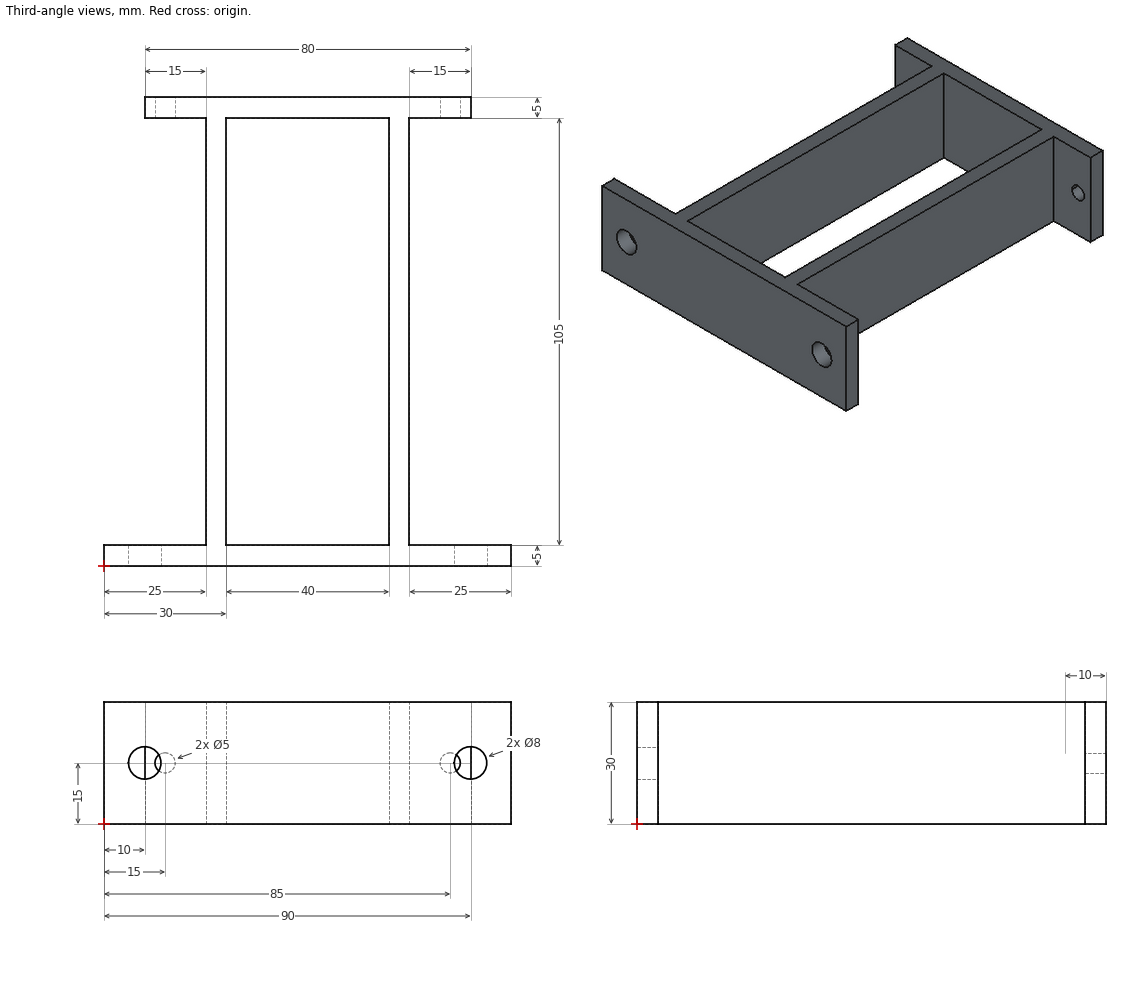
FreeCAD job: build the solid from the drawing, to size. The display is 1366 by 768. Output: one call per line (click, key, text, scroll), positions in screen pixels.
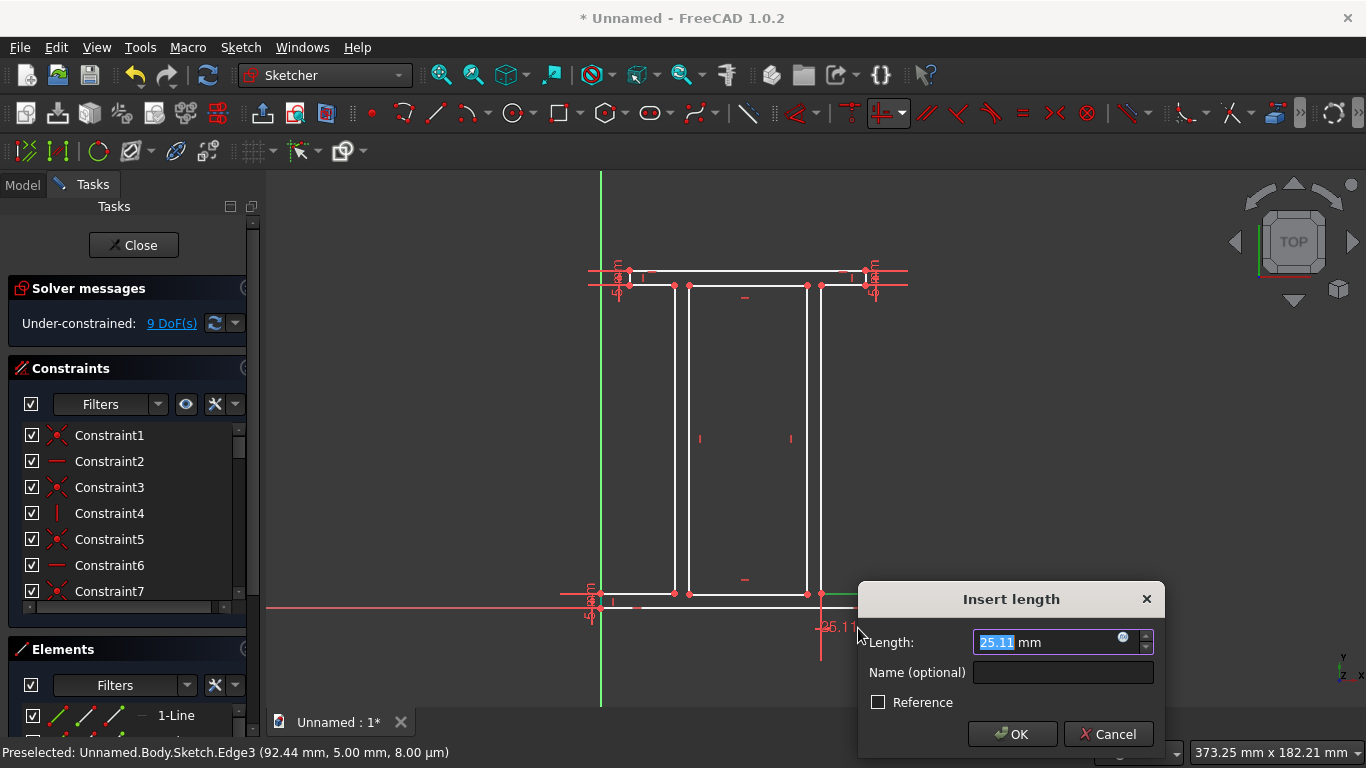
text(25)
key(Return)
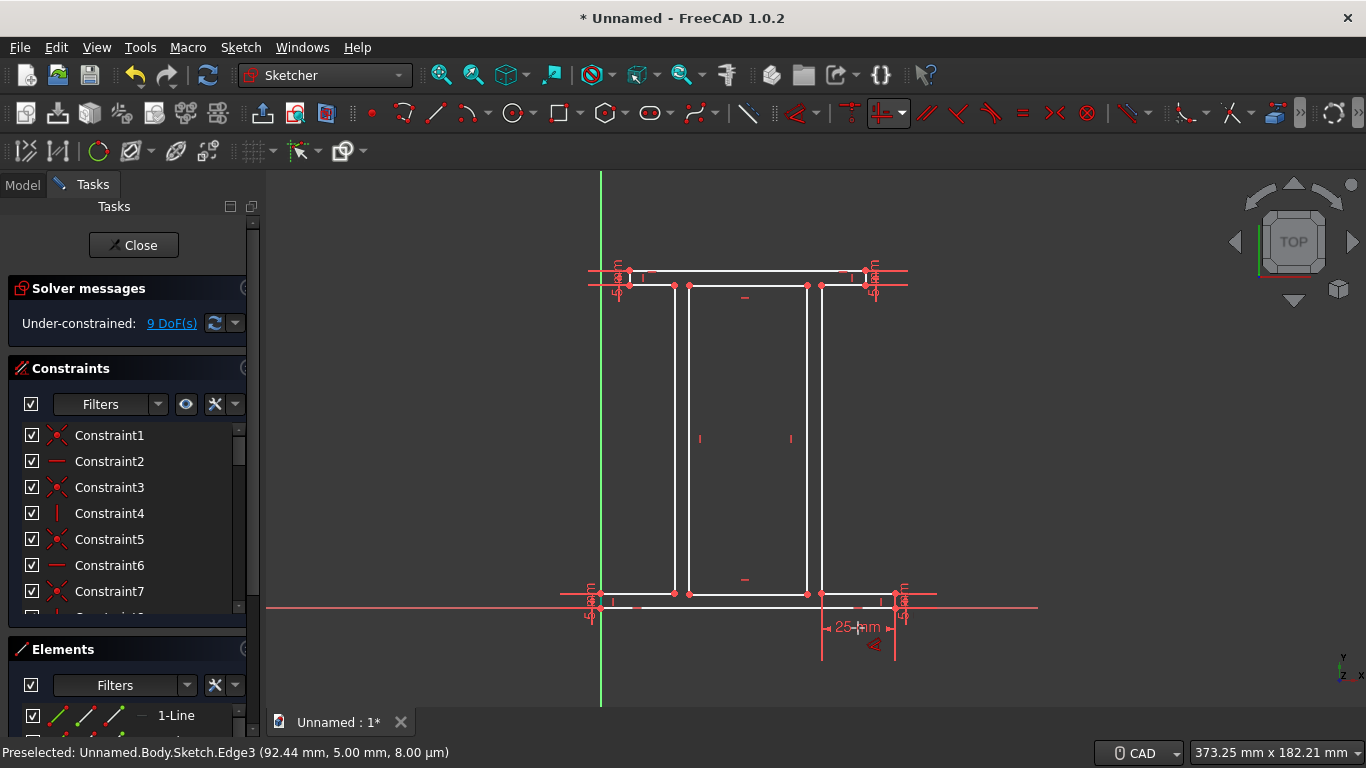
click(835, 285)
click(844, 251)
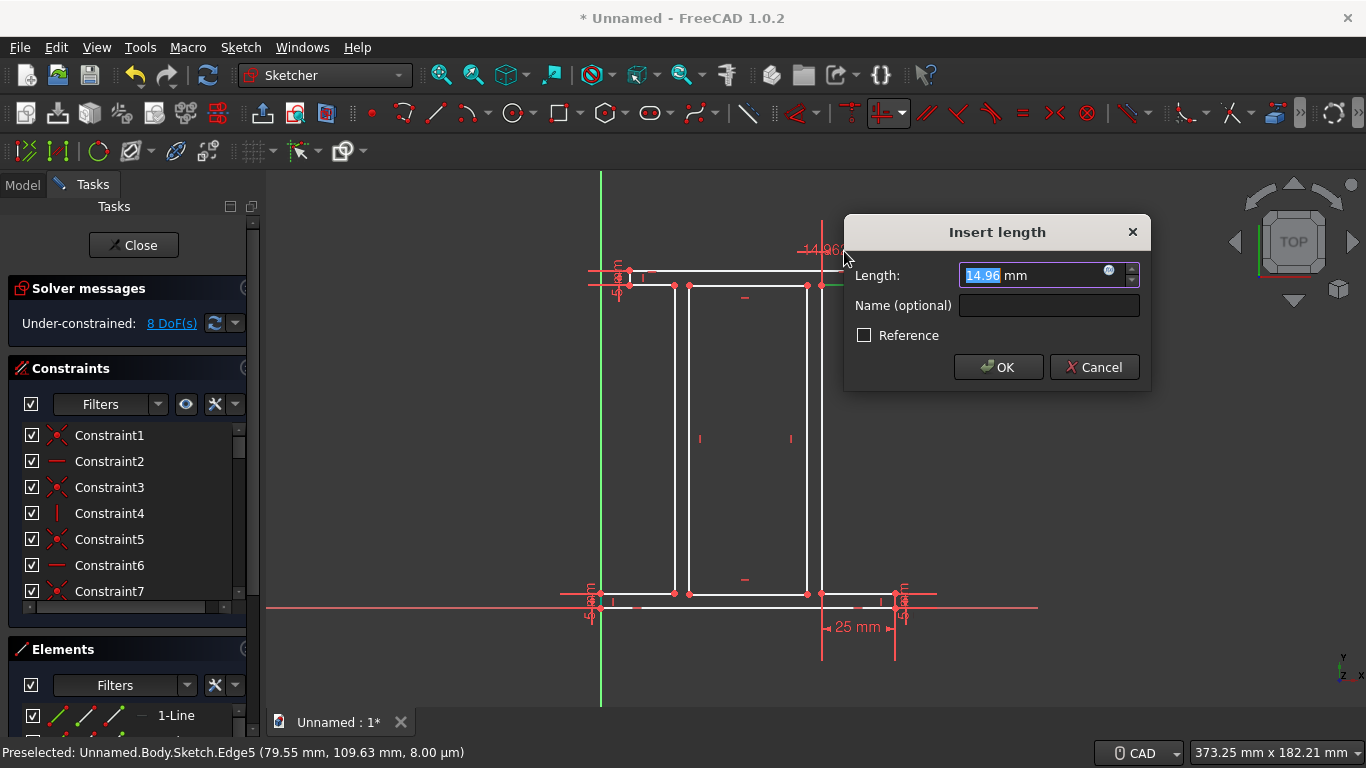
text(15)
key(Return)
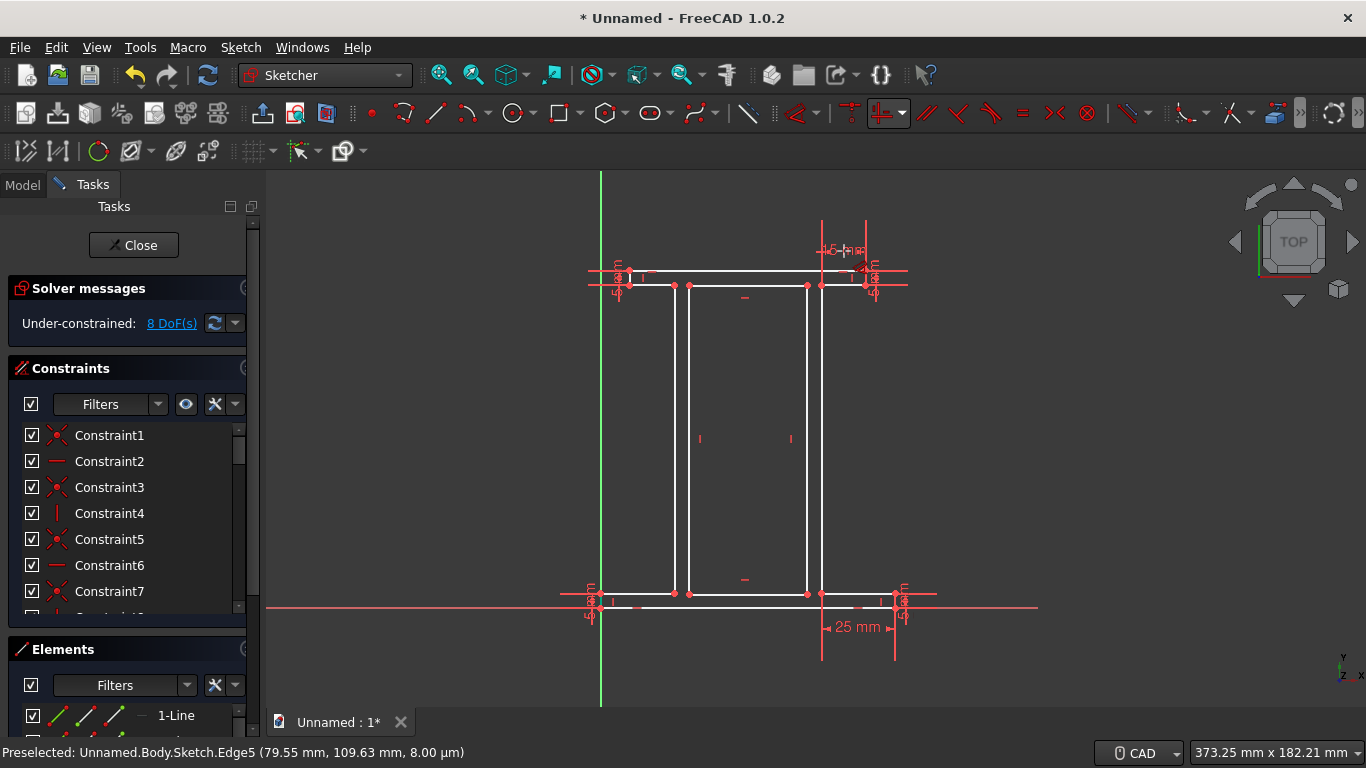
click(795, 271)
click(748, 237)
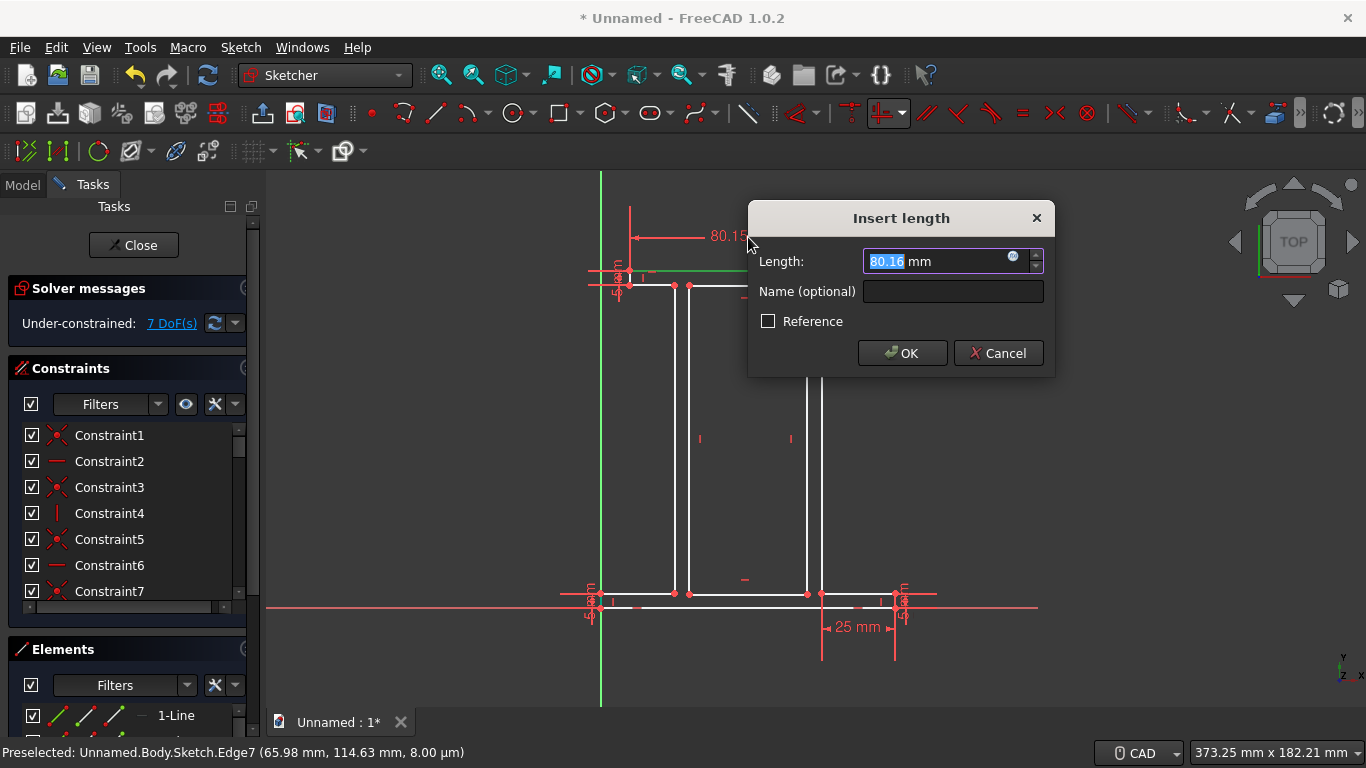
text(80)
key(Return)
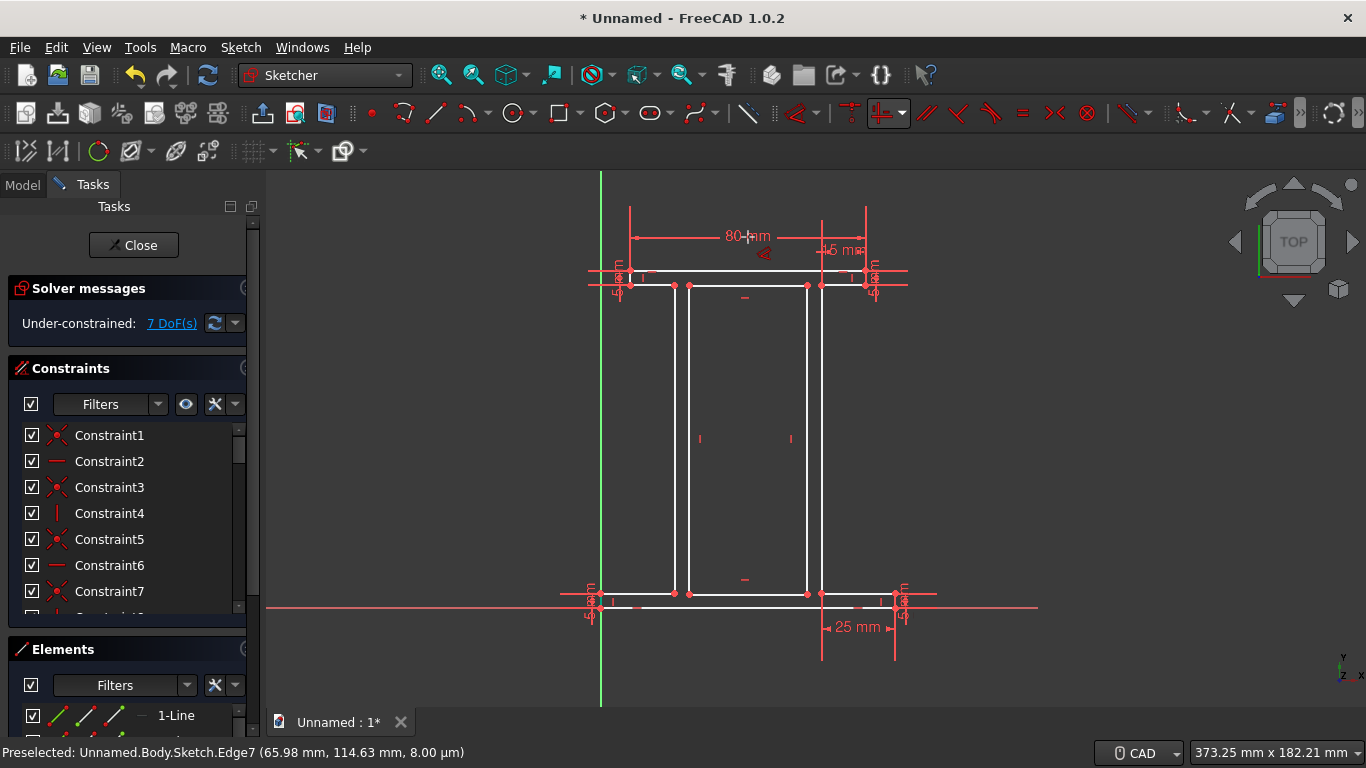
click(643, 285)
click(652, 251)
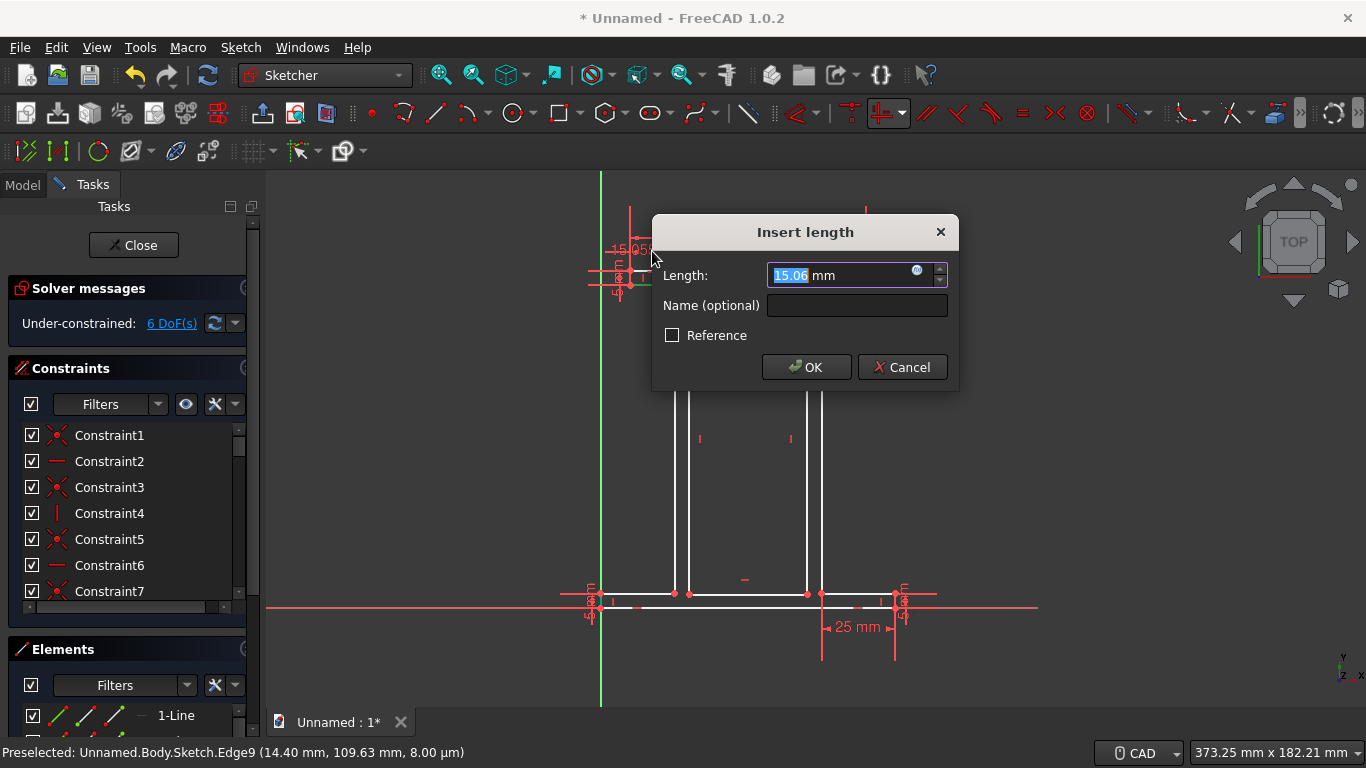
text(15)
key(Return)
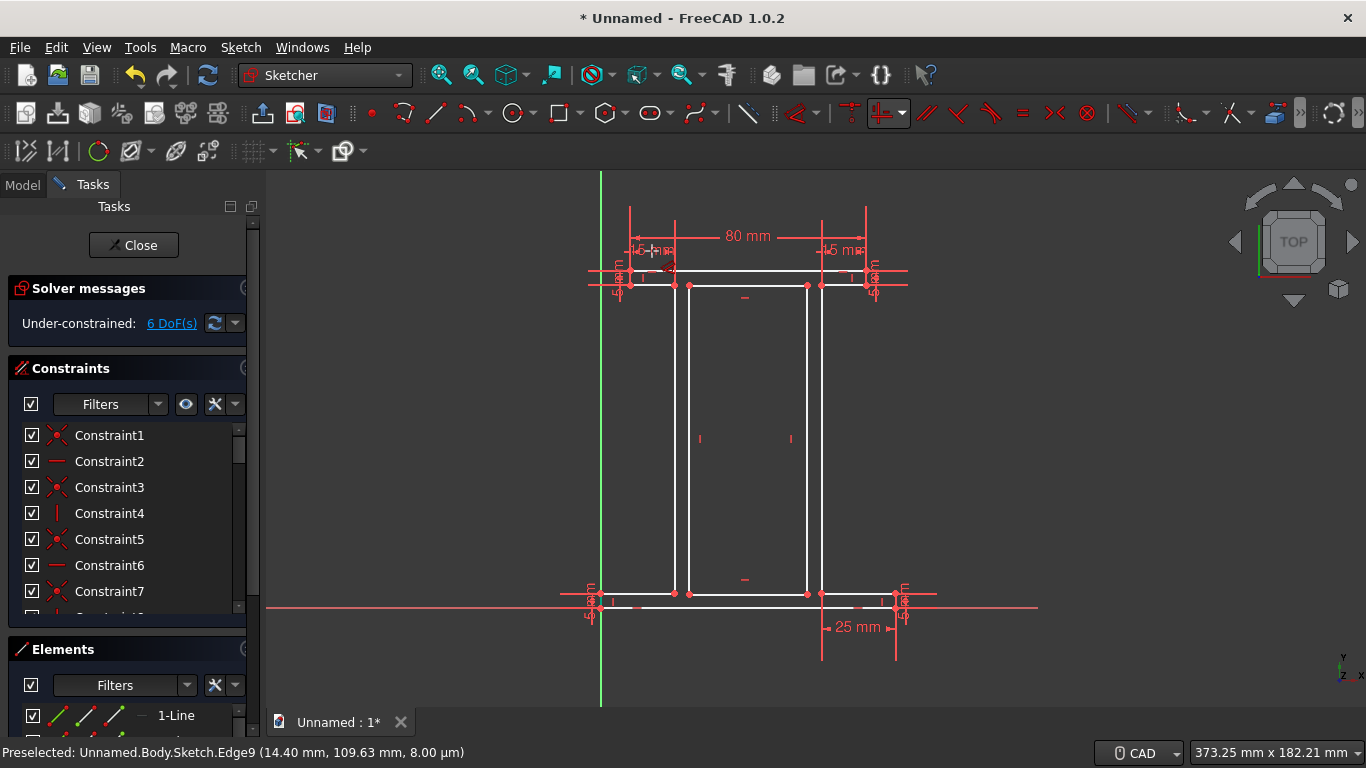
click(652, 594)
click(638, 628)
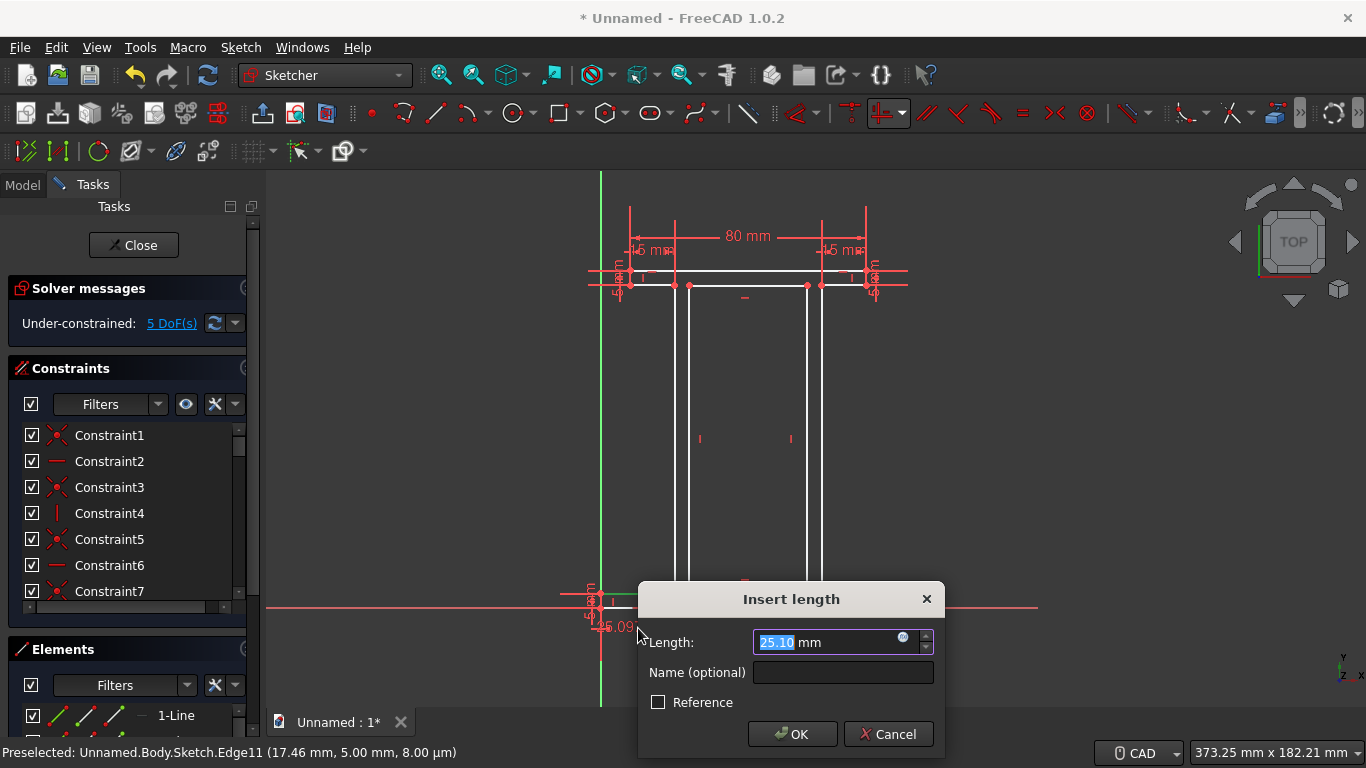
text(25)
key(Return)